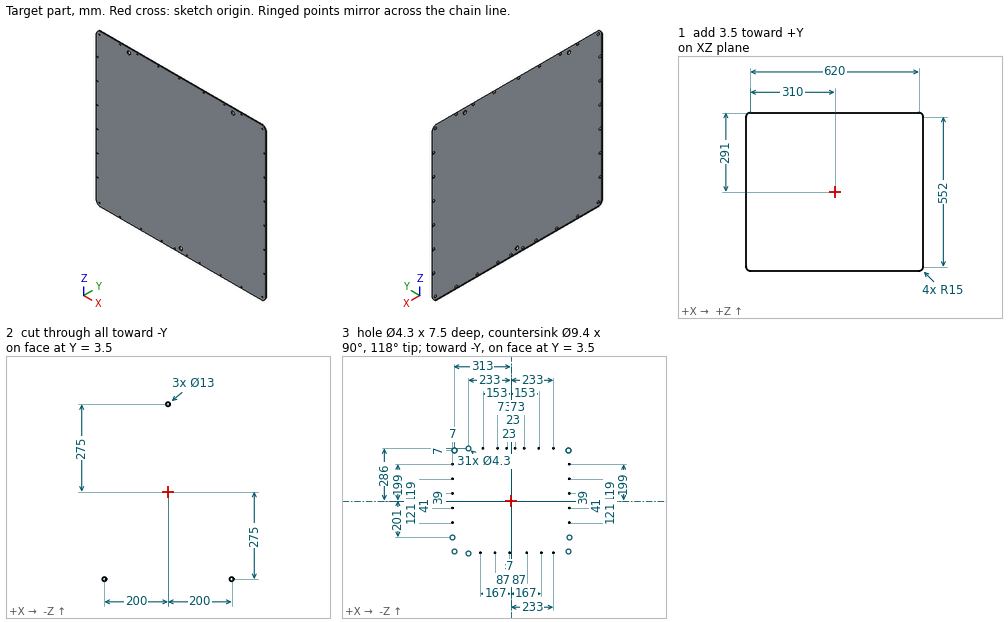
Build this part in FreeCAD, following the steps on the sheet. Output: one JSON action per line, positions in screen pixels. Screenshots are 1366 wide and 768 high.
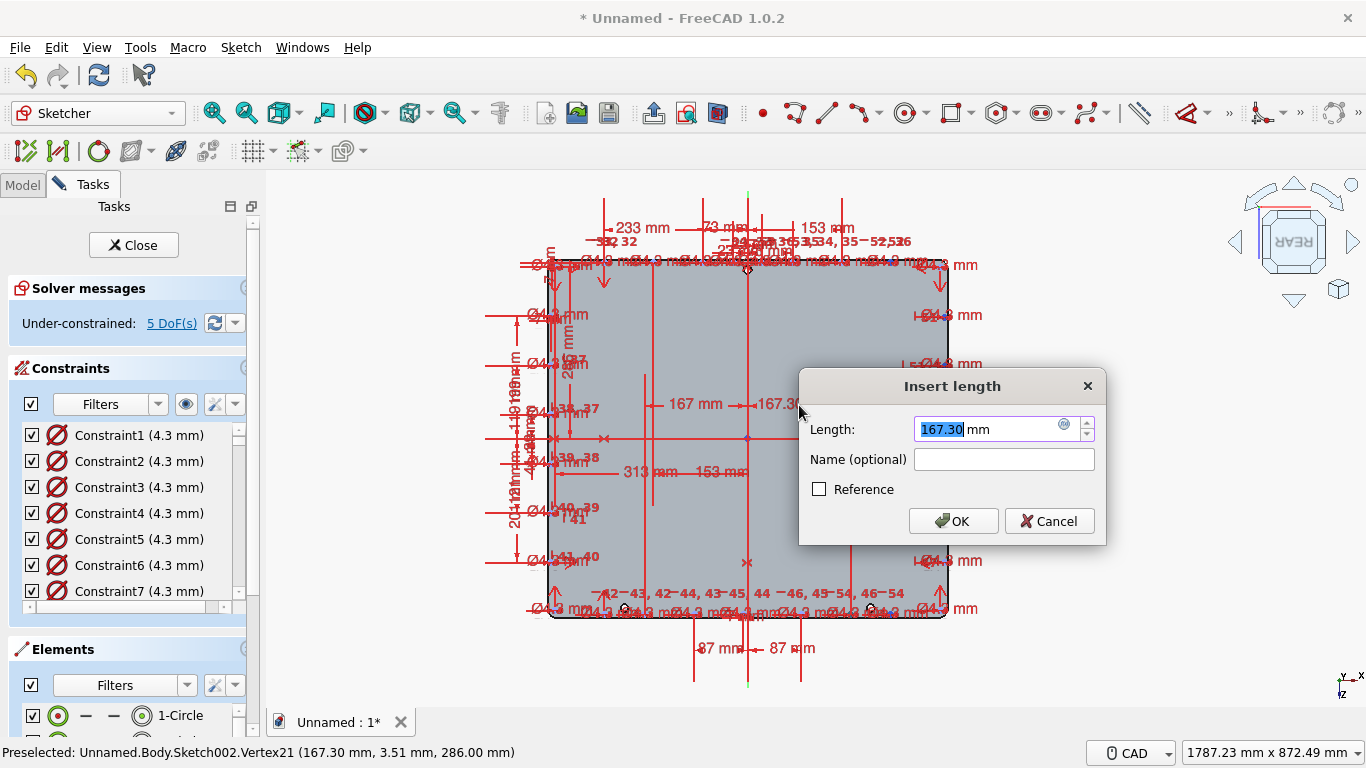
{"action": "type", "text": "167"}
{"action": "key", "text": "Return"}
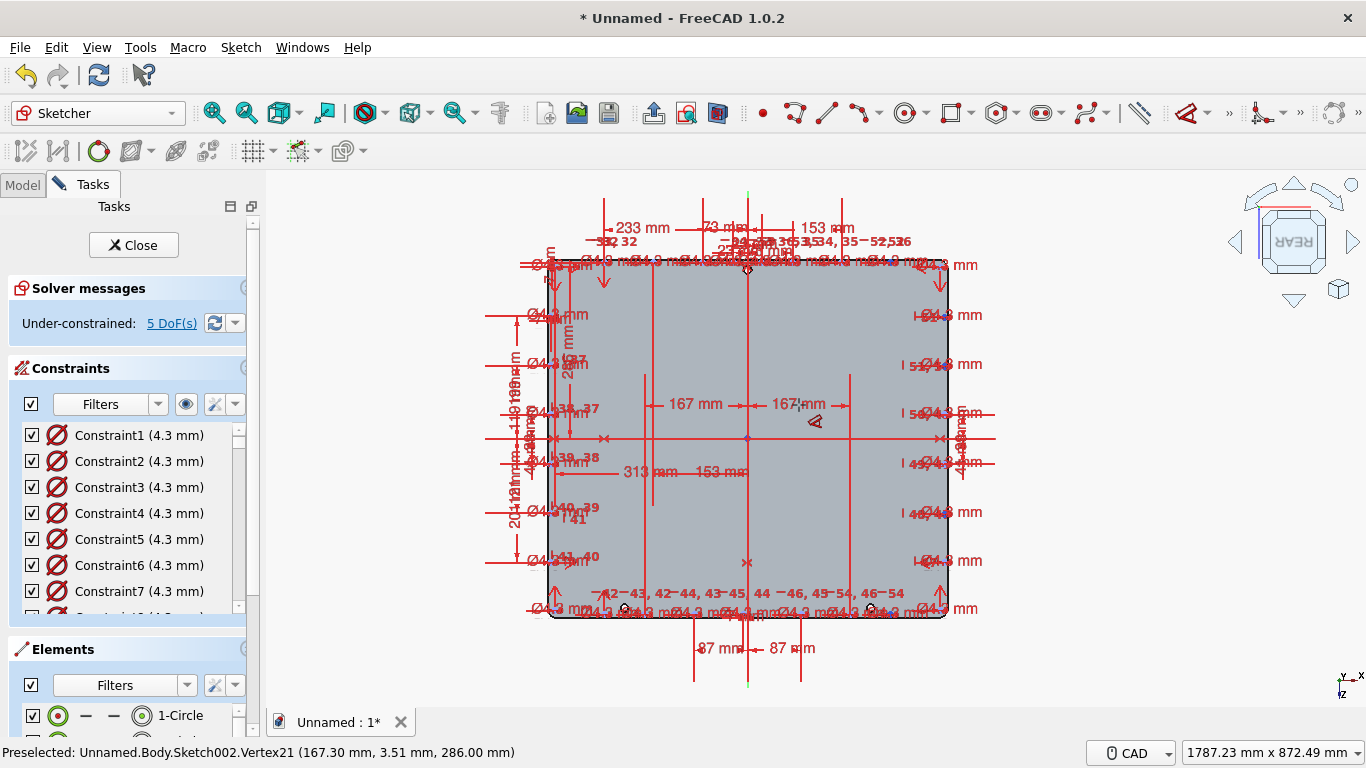
{"action": "left_click", "coordinate": [945, 514]}
{"action": "left_click", "coordinate": [979, 477]}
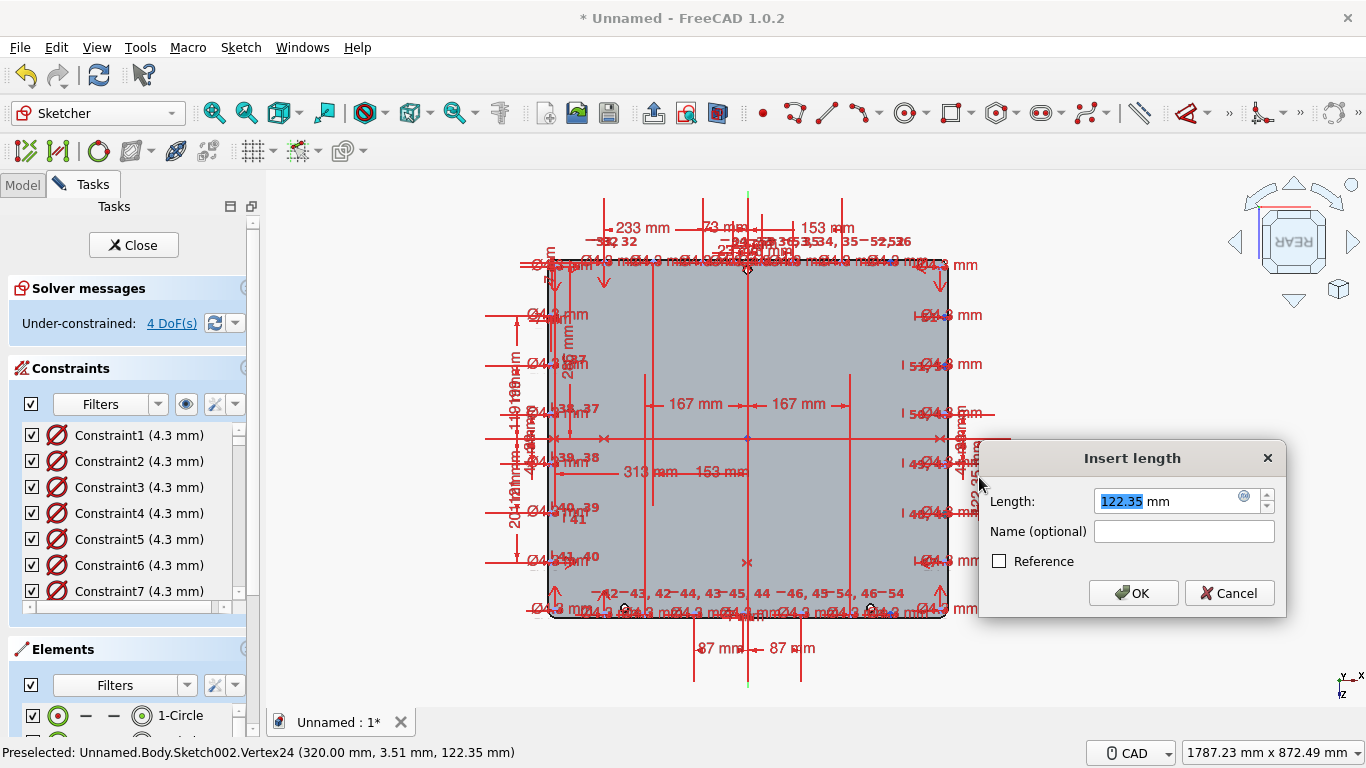
{"action": "type", "text": "121"}
{"action": "key", "text": "Return"}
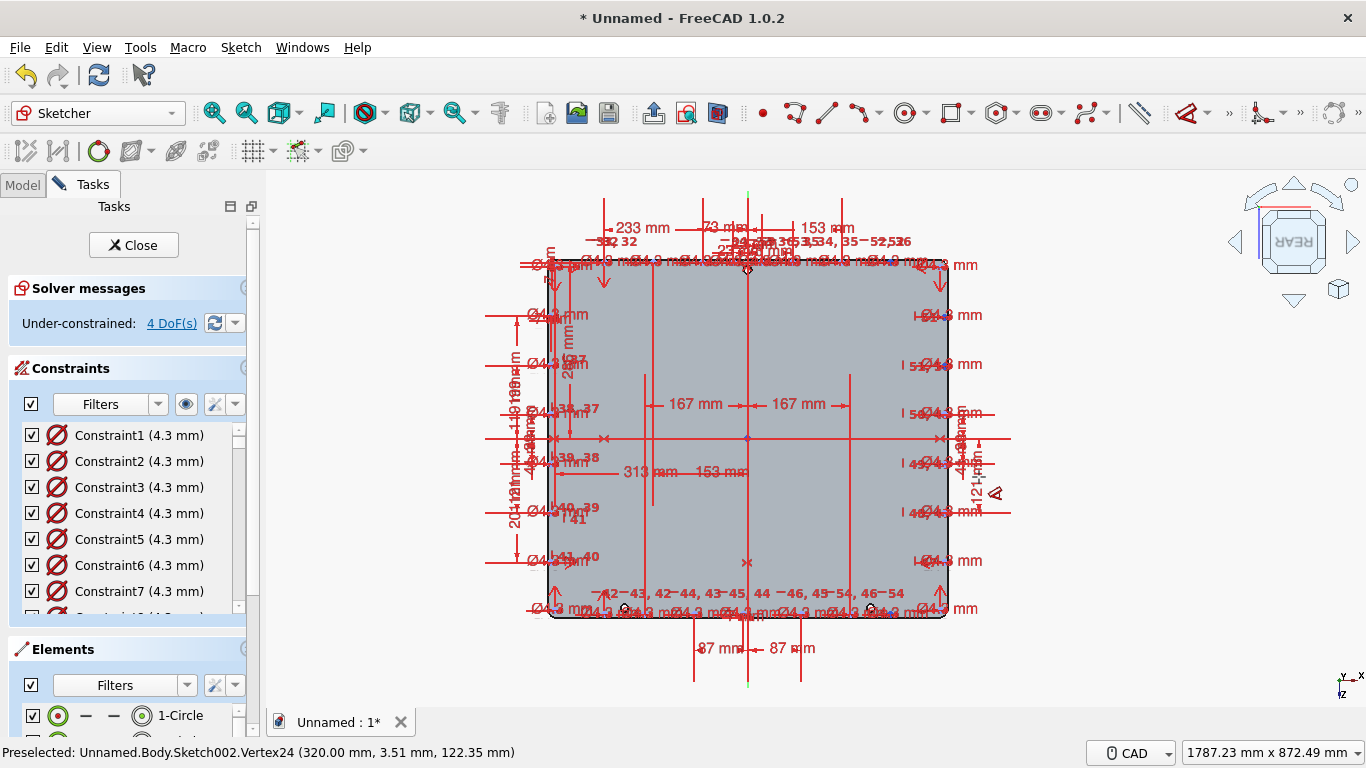
{"action": "left_click", "coordinate": [945, 366]}
{"action": "left_click", "coordinate": [979, 403]}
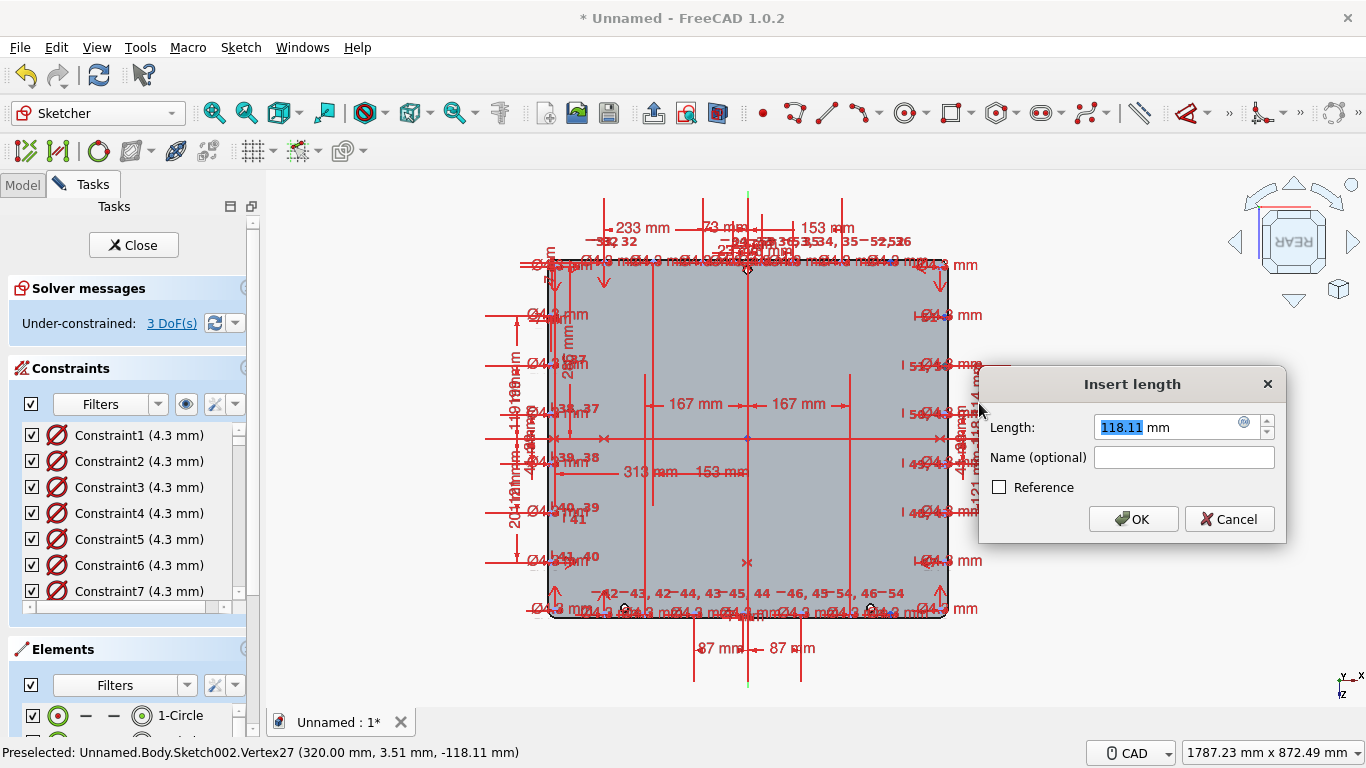
{"action": "type", "text": "119"}
{"action": "key", "text": "Return"}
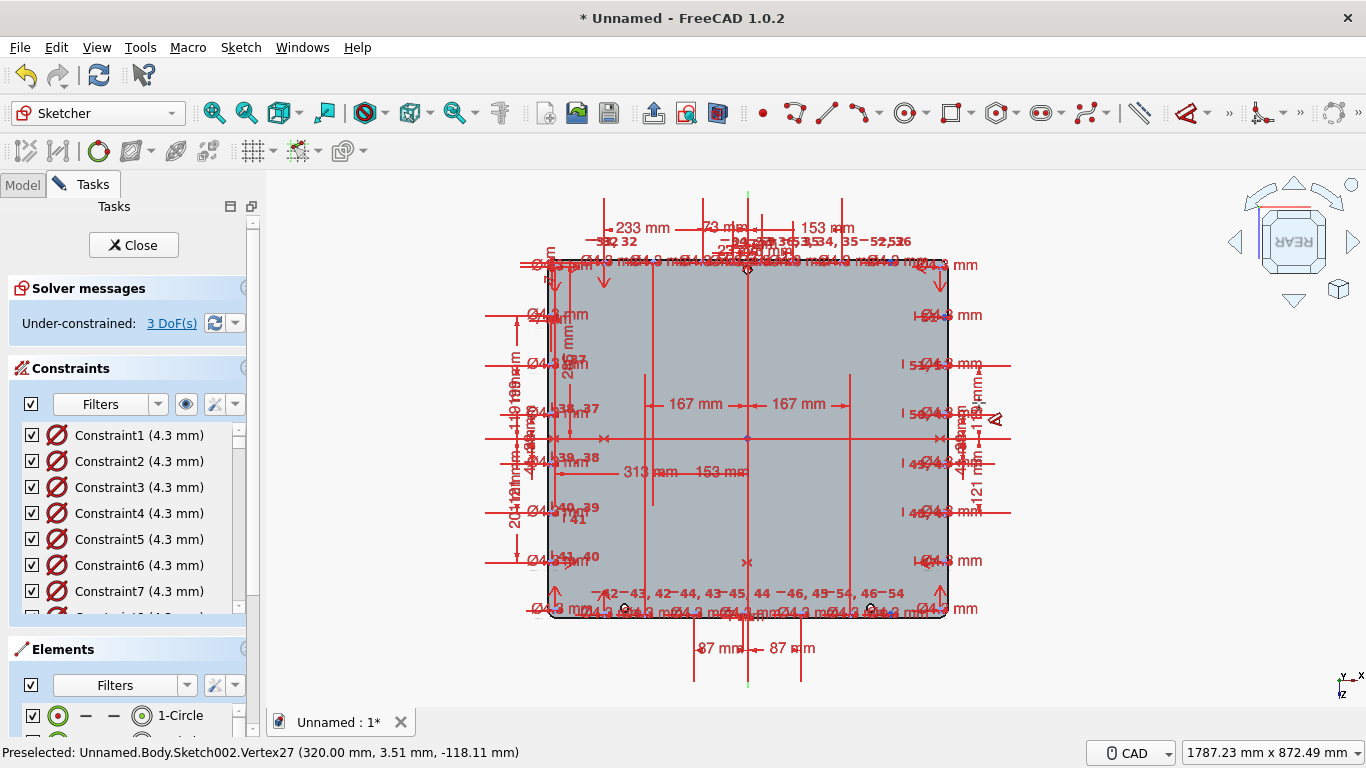
{"action": "left_click", "coordinate": [945, 317]}
{"action": "left_click", "coordinate": [979, 378]}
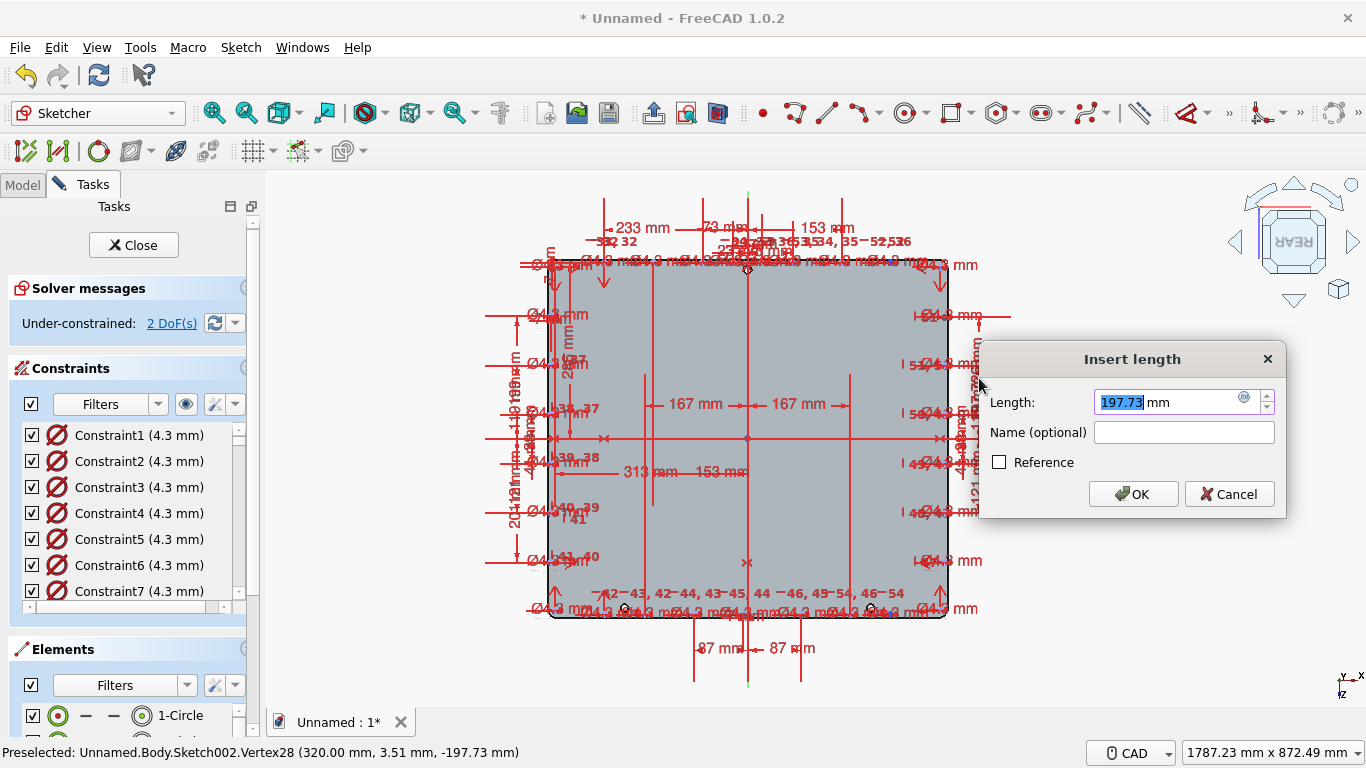
{"action": "type", "text": "199"}
{"action": "key", "text": "Return"}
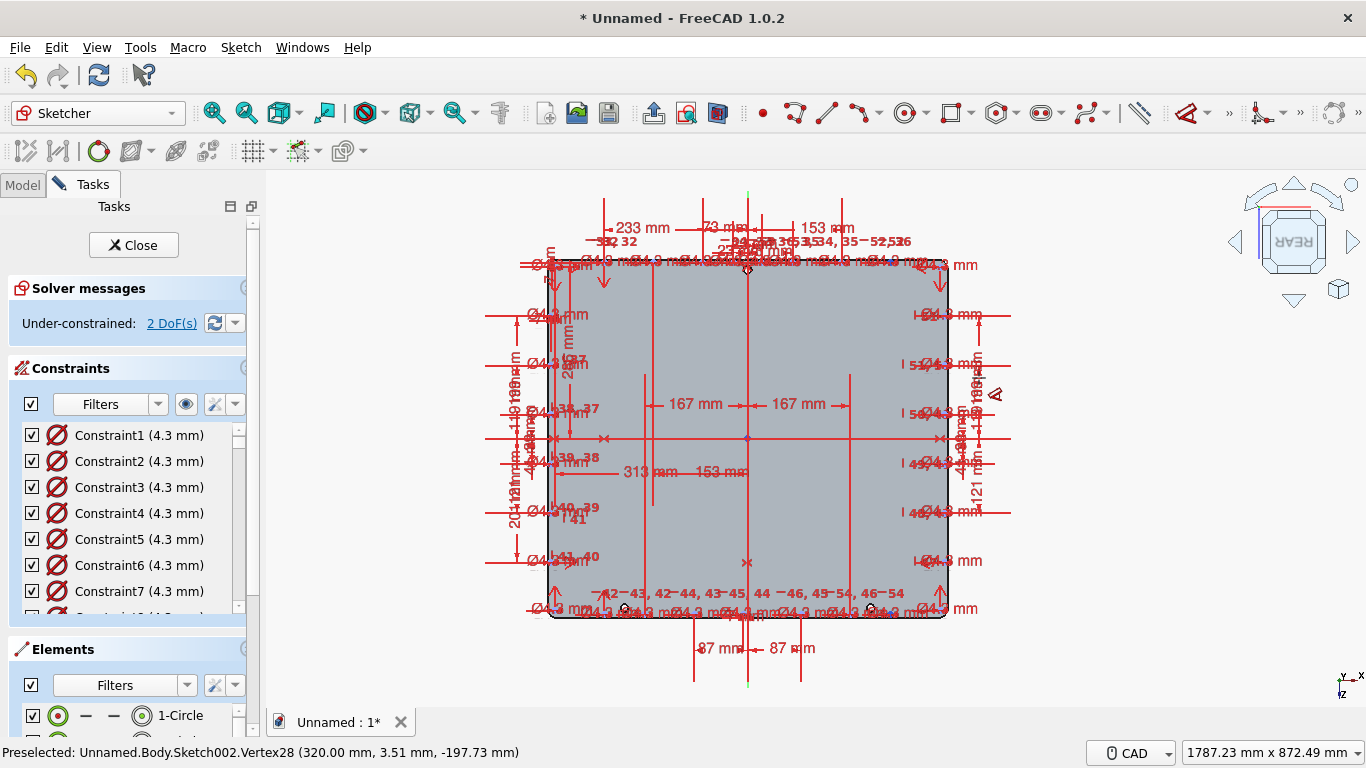
{"action": "left_click", "coordinate": [891, 263]}
{"action": "left_click", "coordinate": [819, 473]}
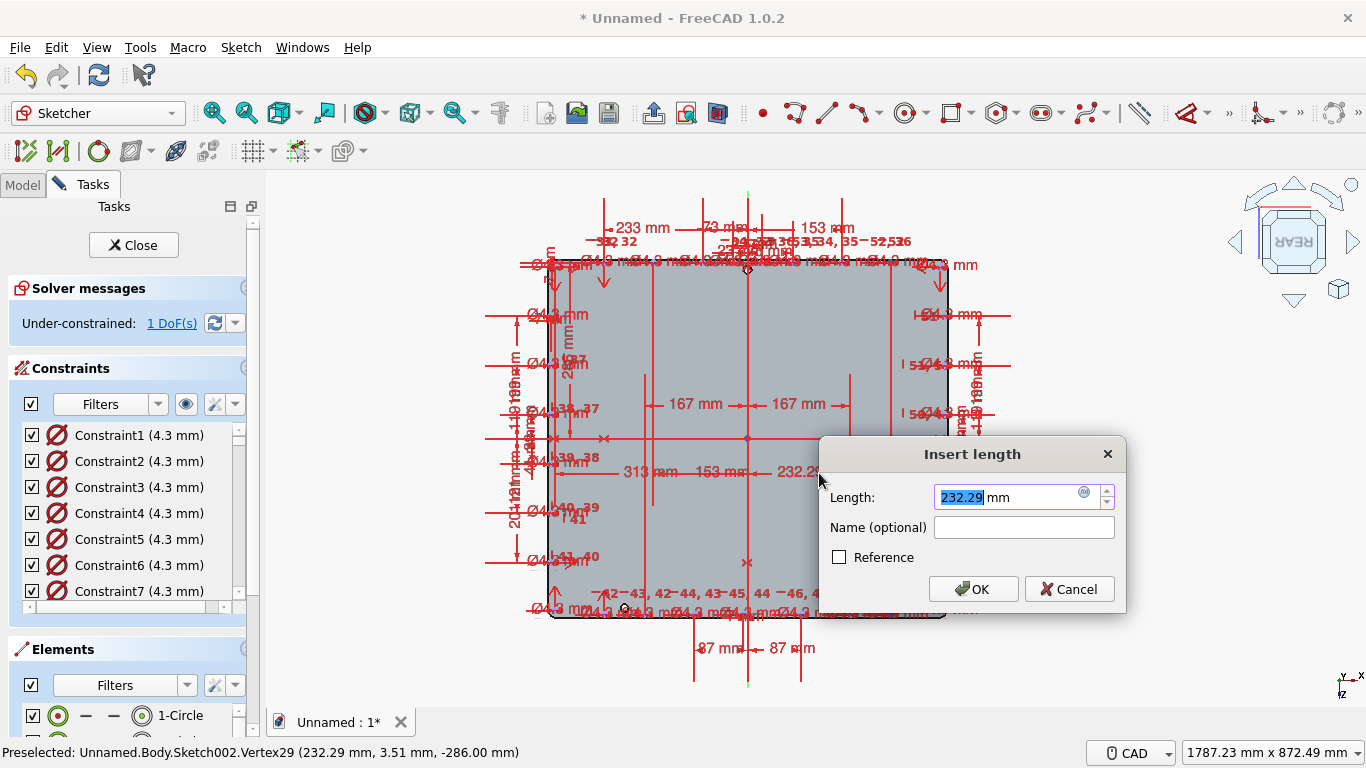
{"action": "type", "text": "233"}
{"action": "key", "text": "Return"}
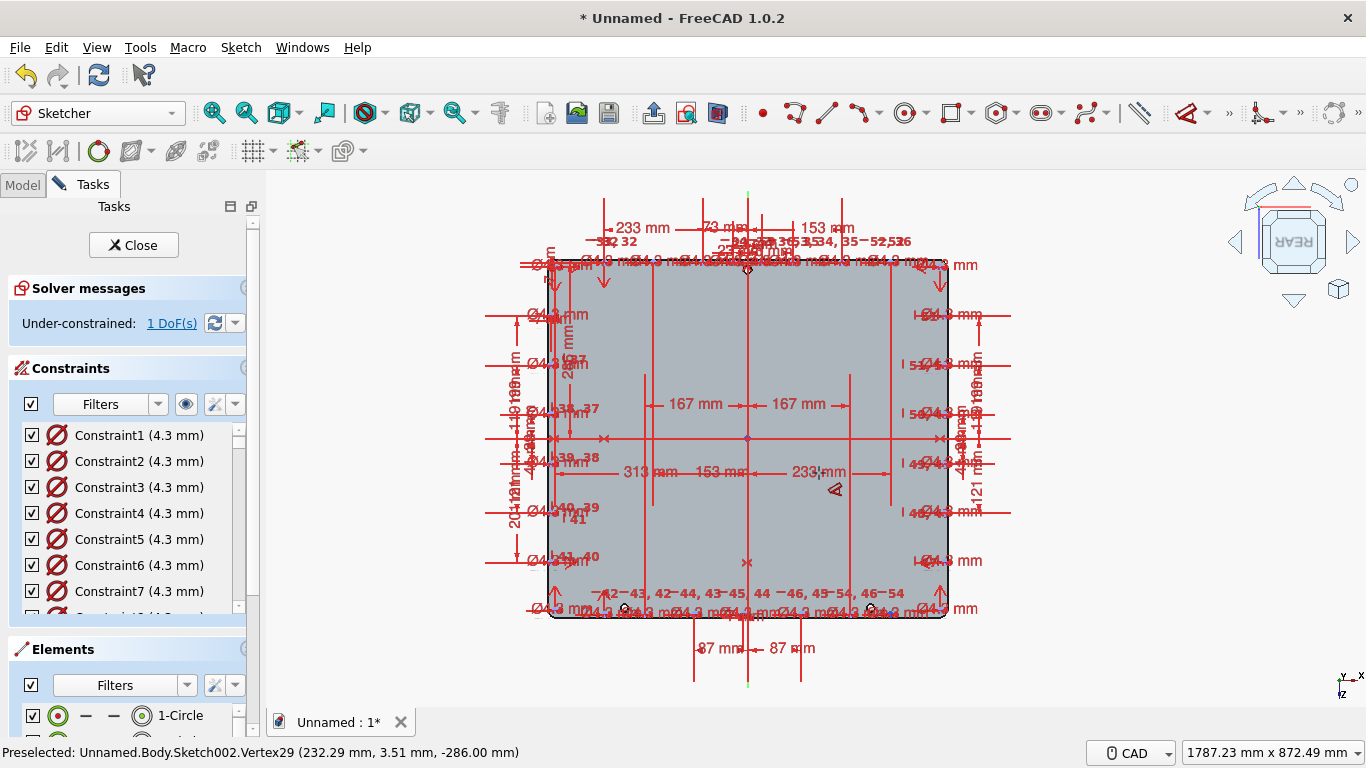
{"action": "left_click", "coordinate": [891, 615]}
{"action": "left_click", "coordinate": [869, 649]}